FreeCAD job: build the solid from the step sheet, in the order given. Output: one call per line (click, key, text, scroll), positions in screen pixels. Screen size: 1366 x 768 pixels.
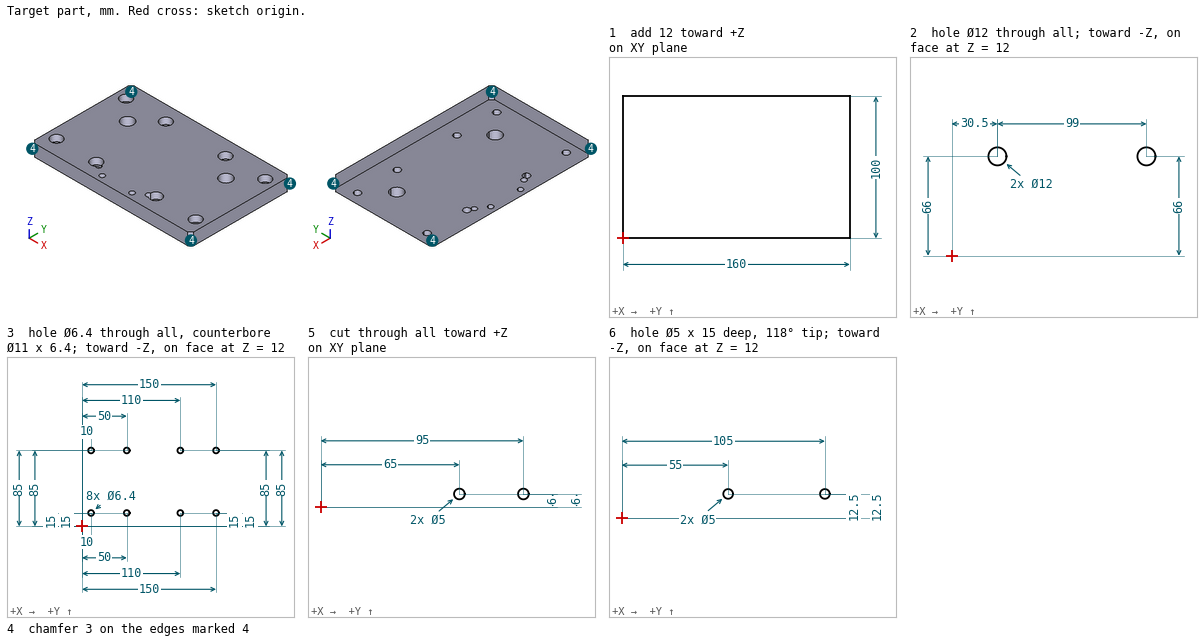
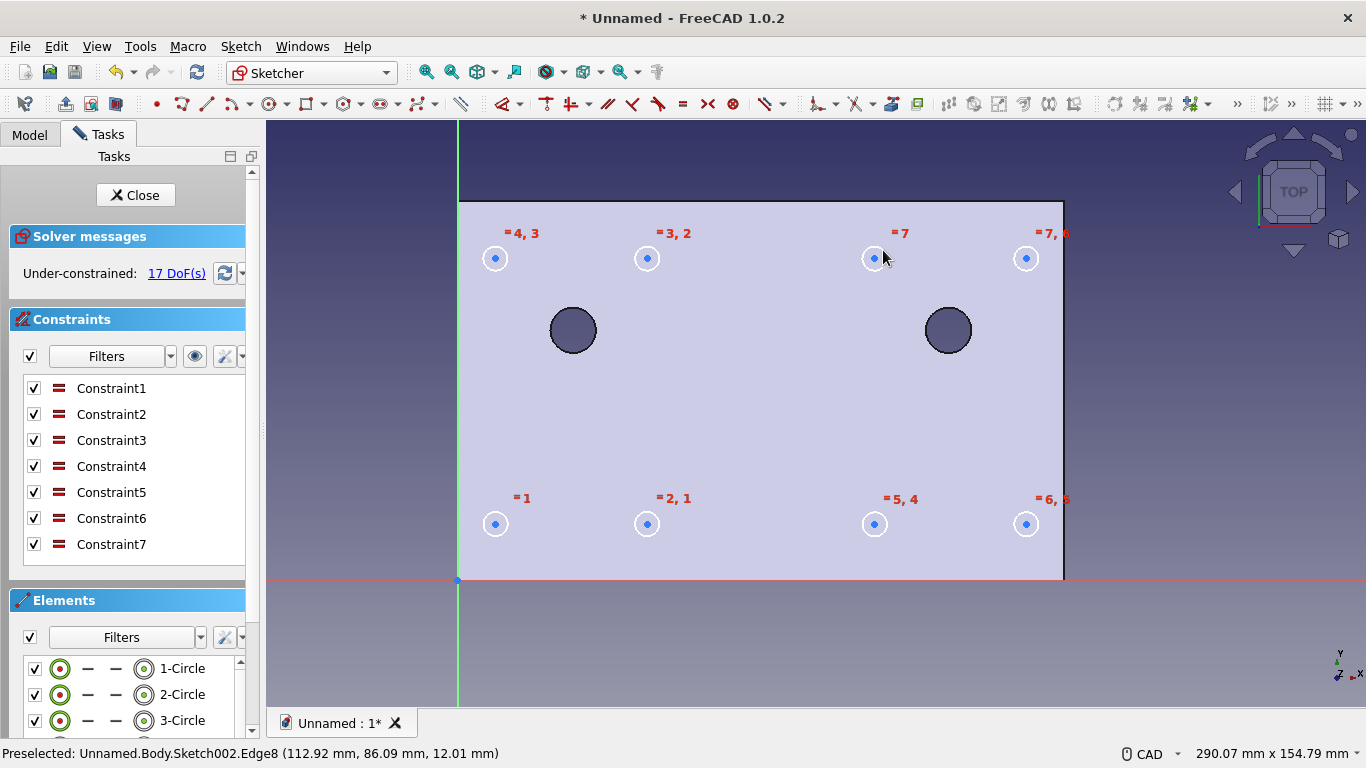
scroll(504, 515, up, 3)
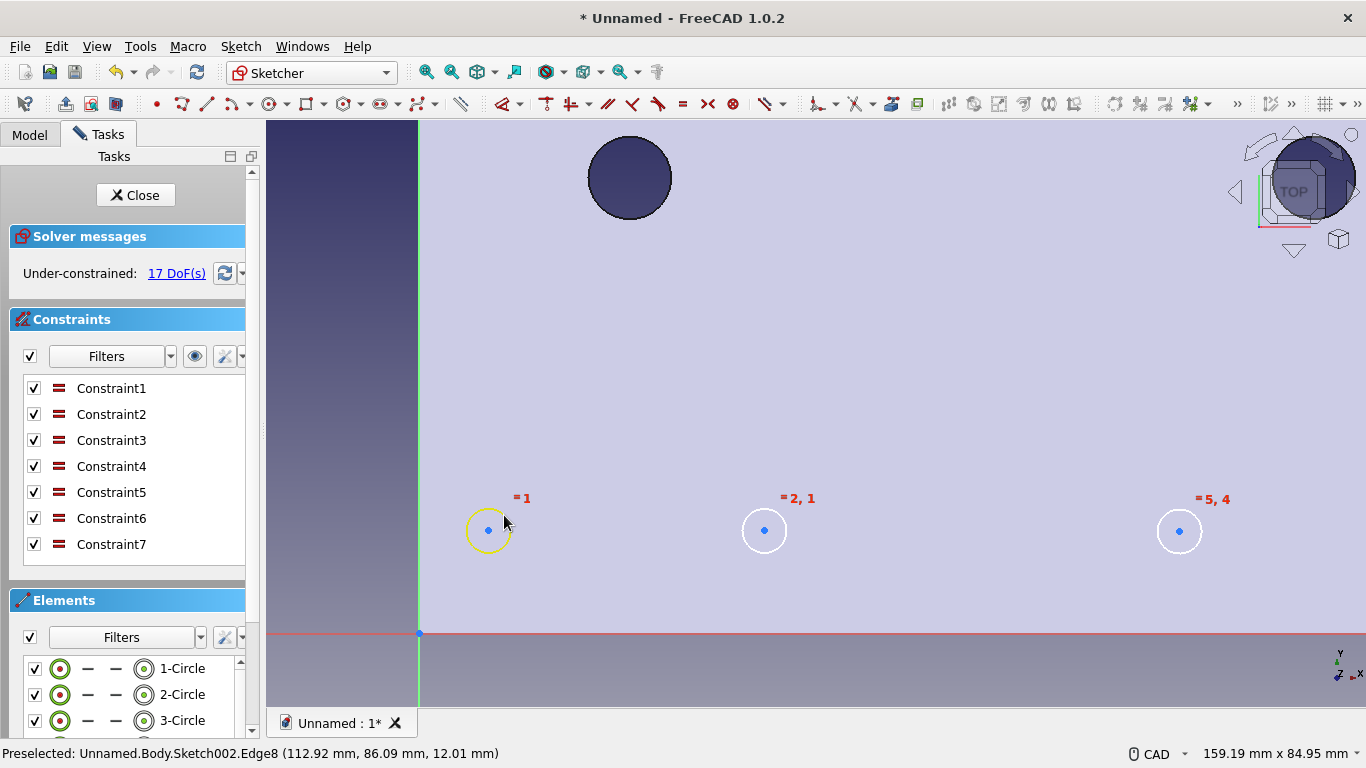
click(504, 515)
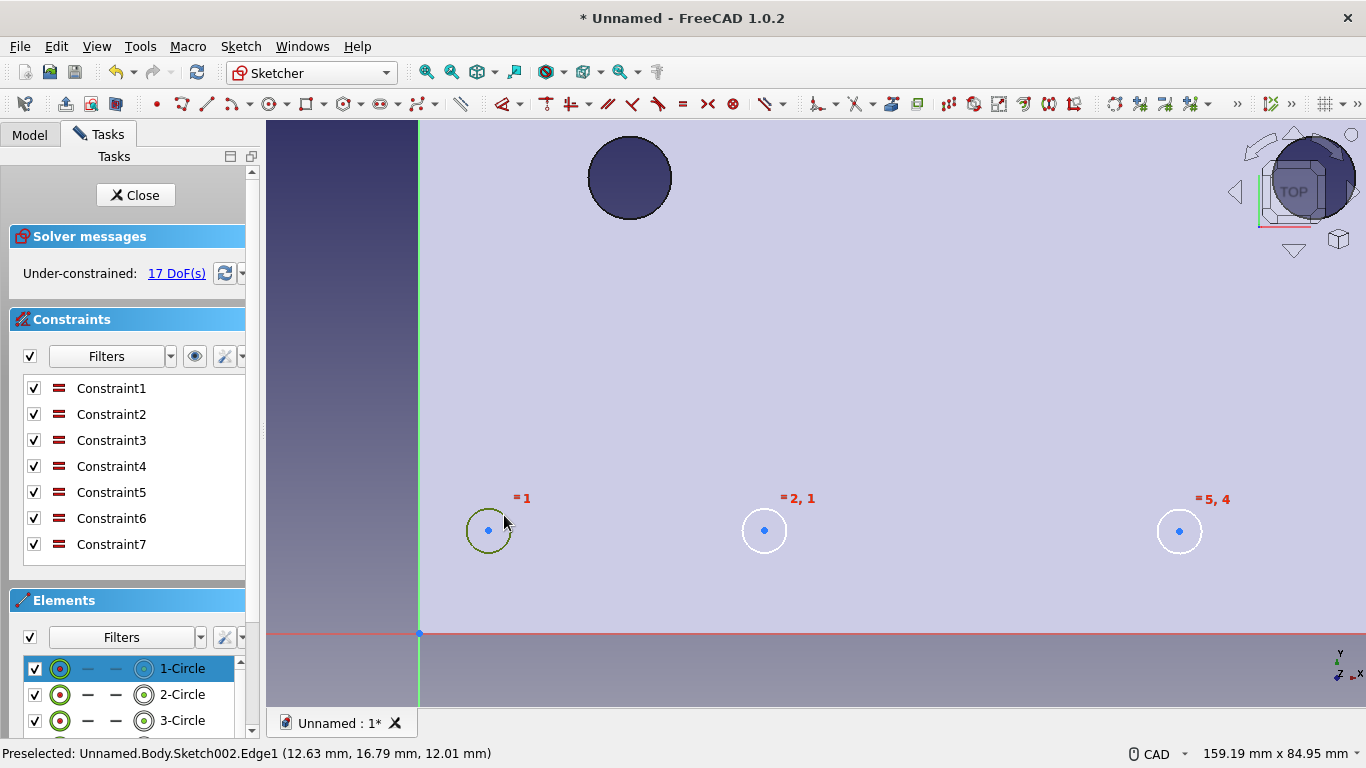
click(520, 104)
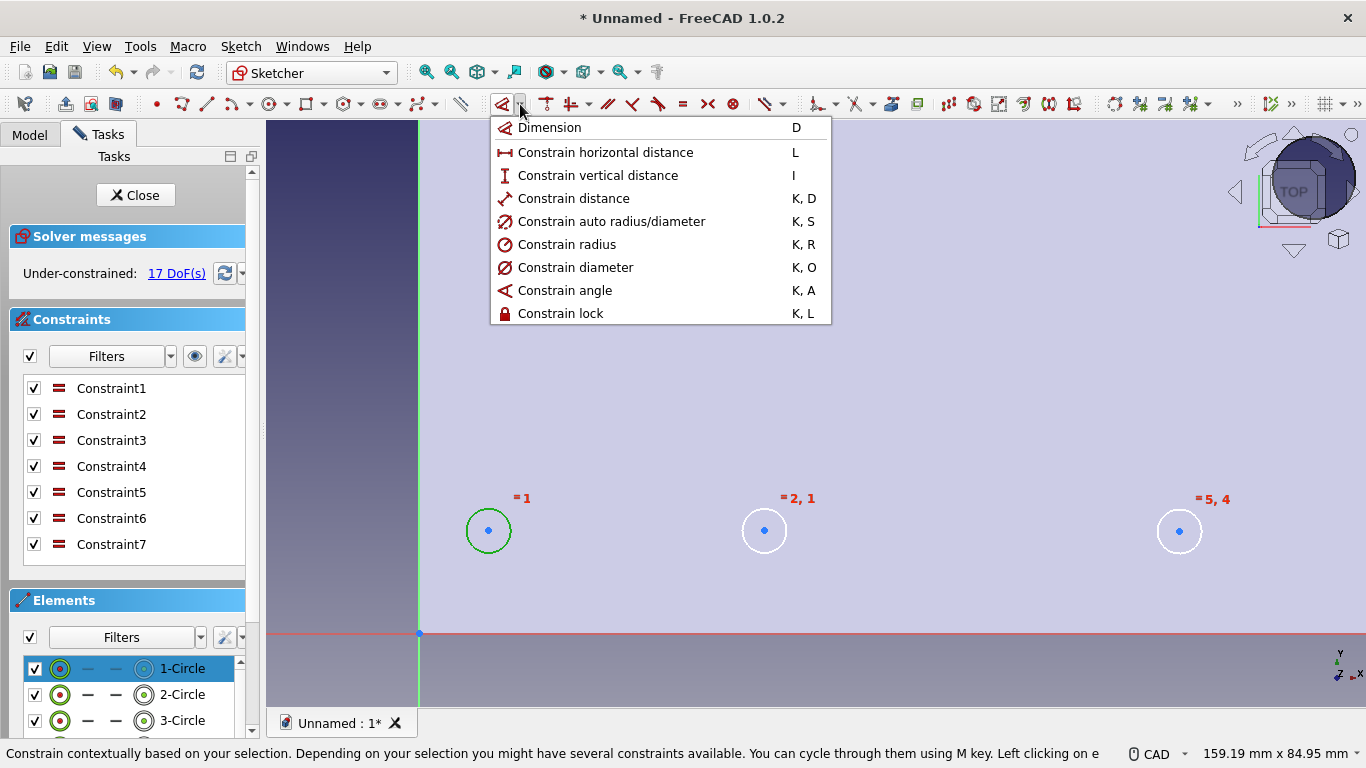
click(661, 268)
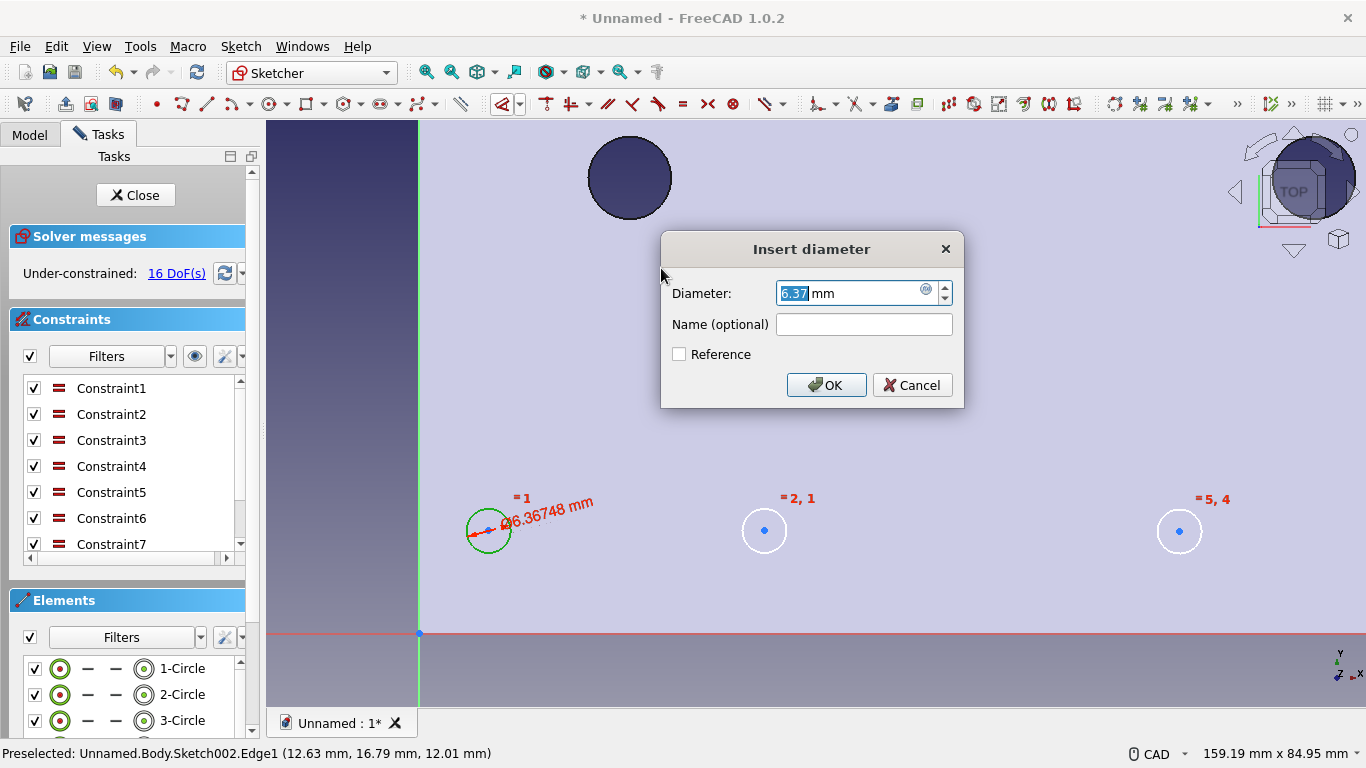
text(6.4)
key(Return)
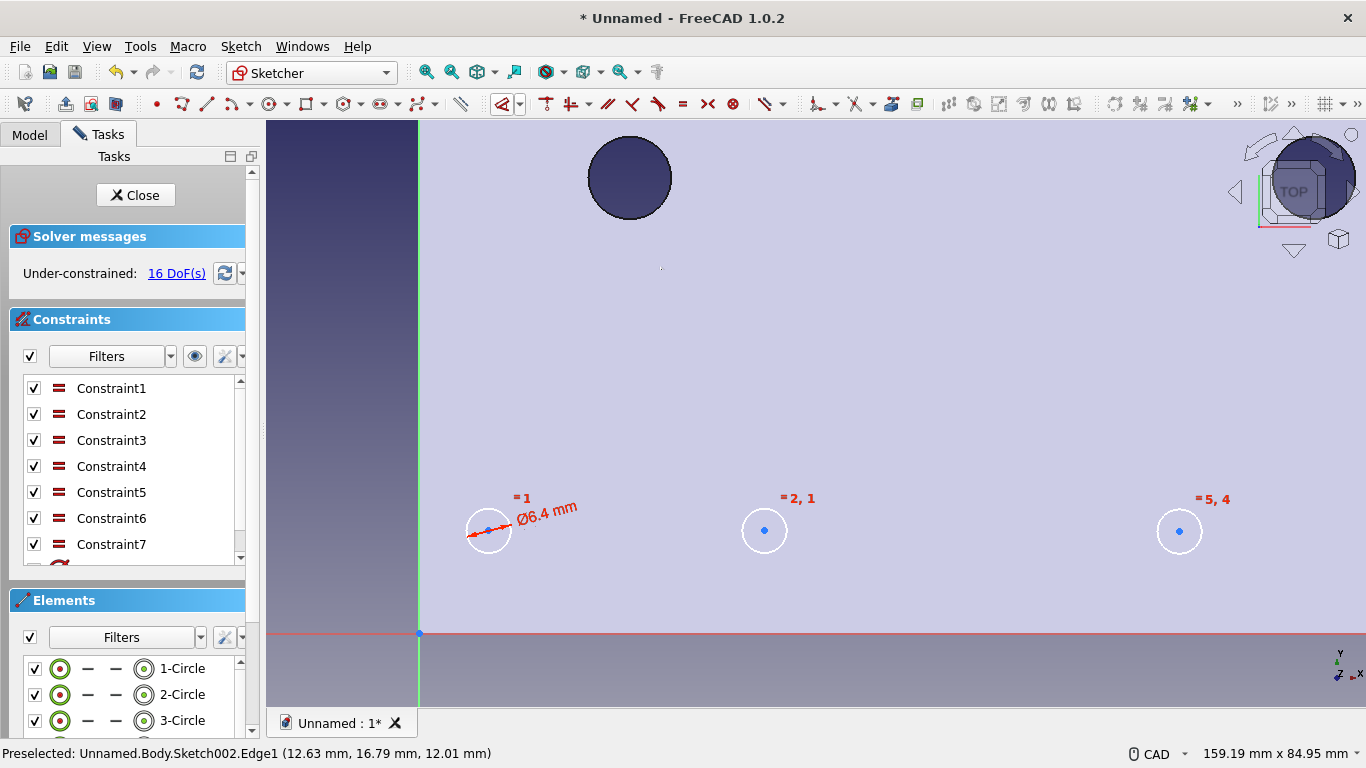
click(489, 531)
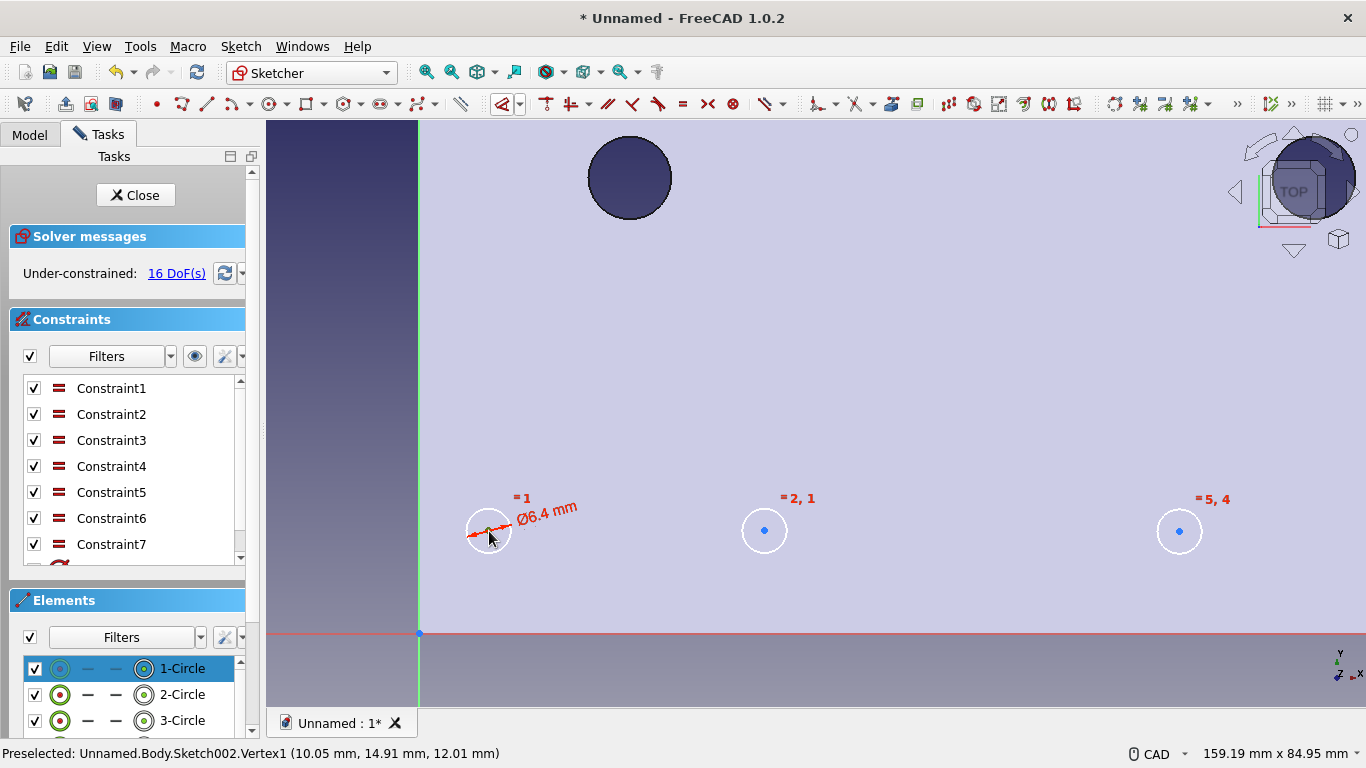
key(l)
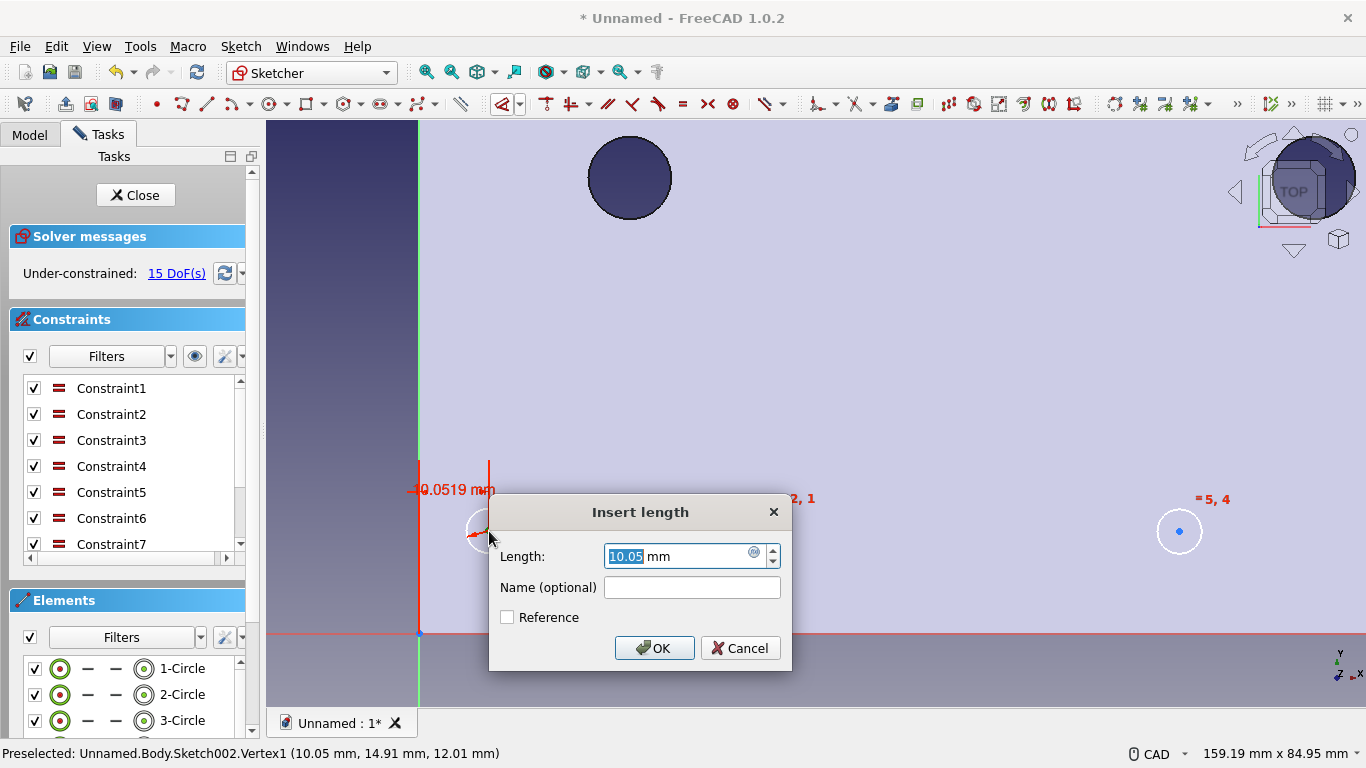
text(10)
key(Return)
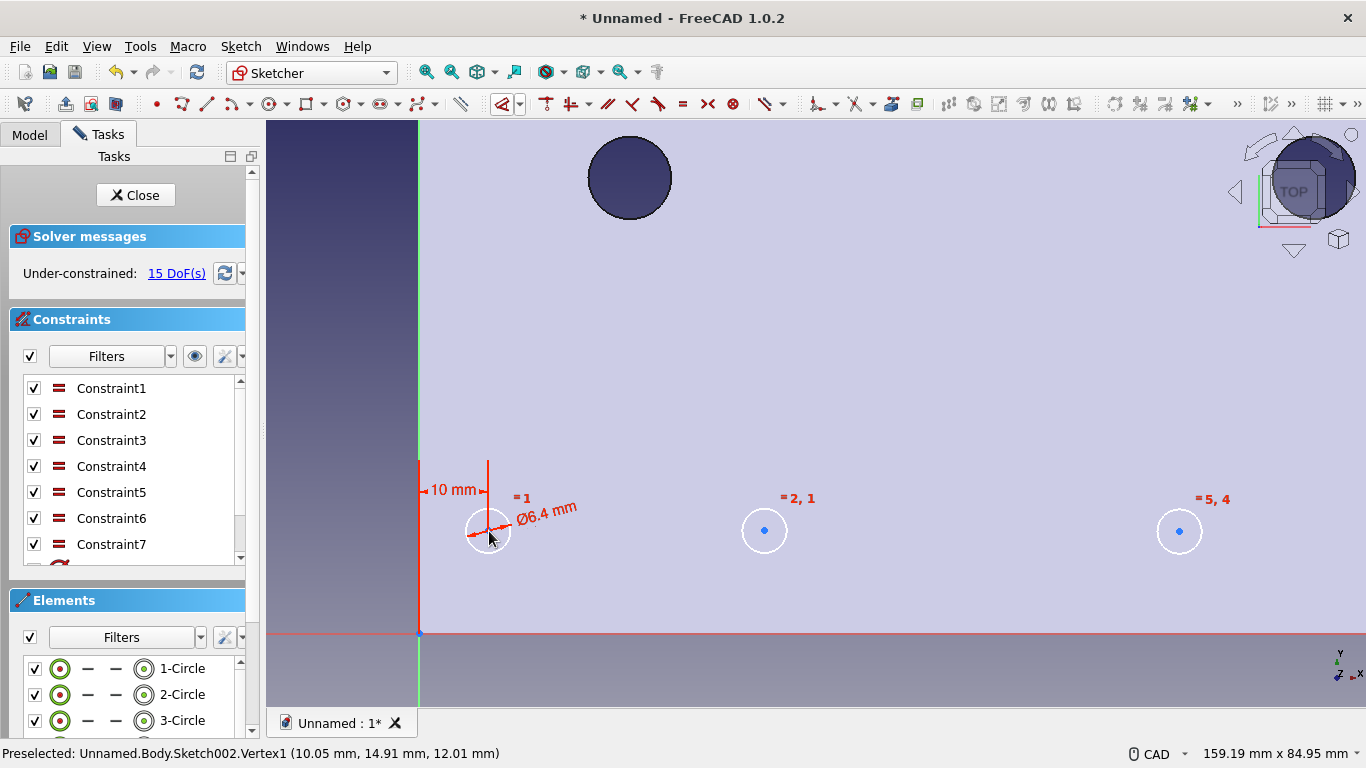
click(488, 531)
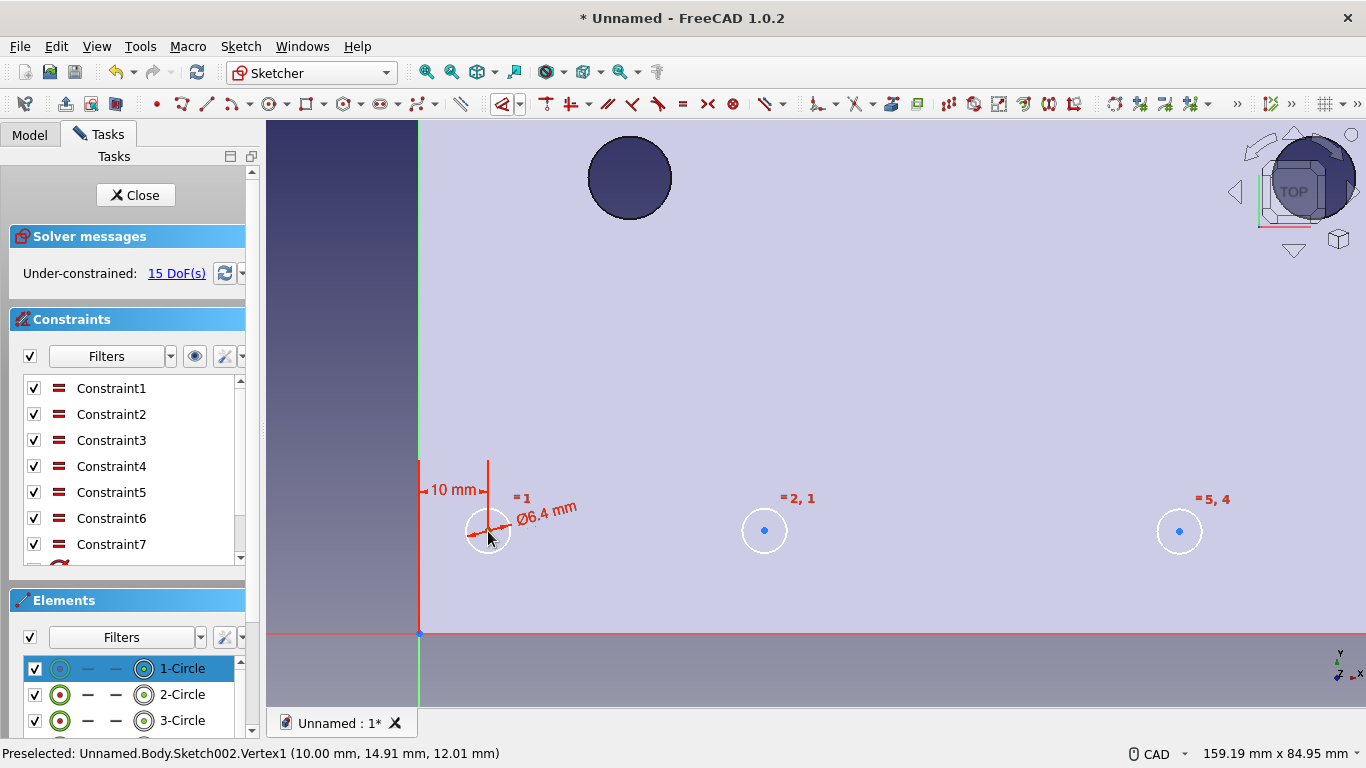
key(i)